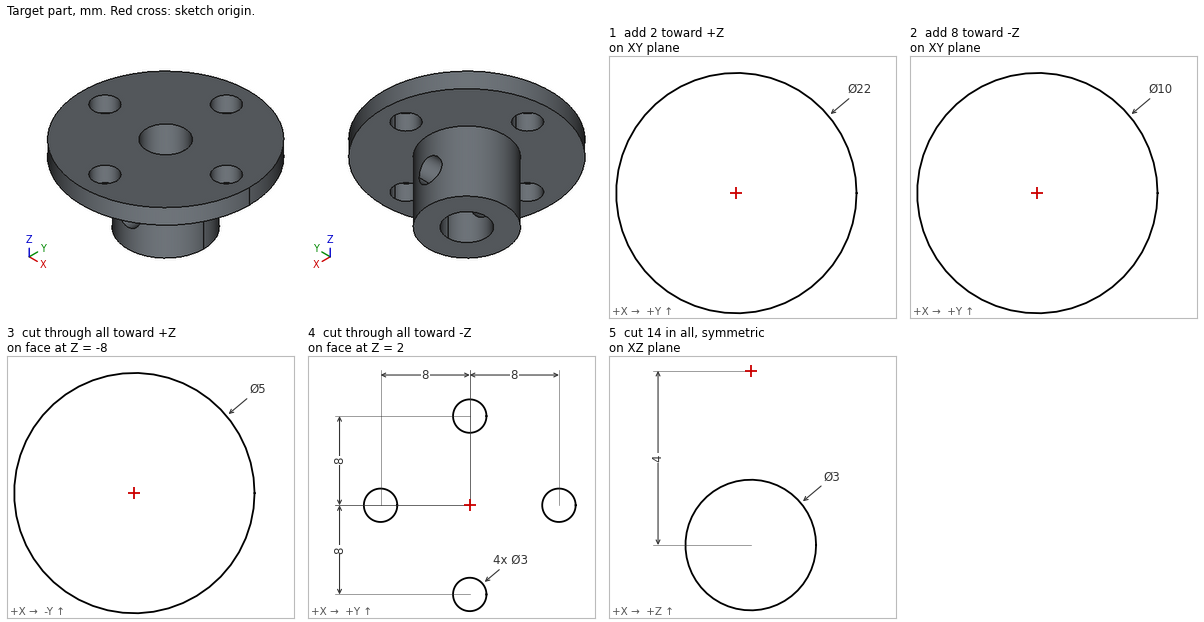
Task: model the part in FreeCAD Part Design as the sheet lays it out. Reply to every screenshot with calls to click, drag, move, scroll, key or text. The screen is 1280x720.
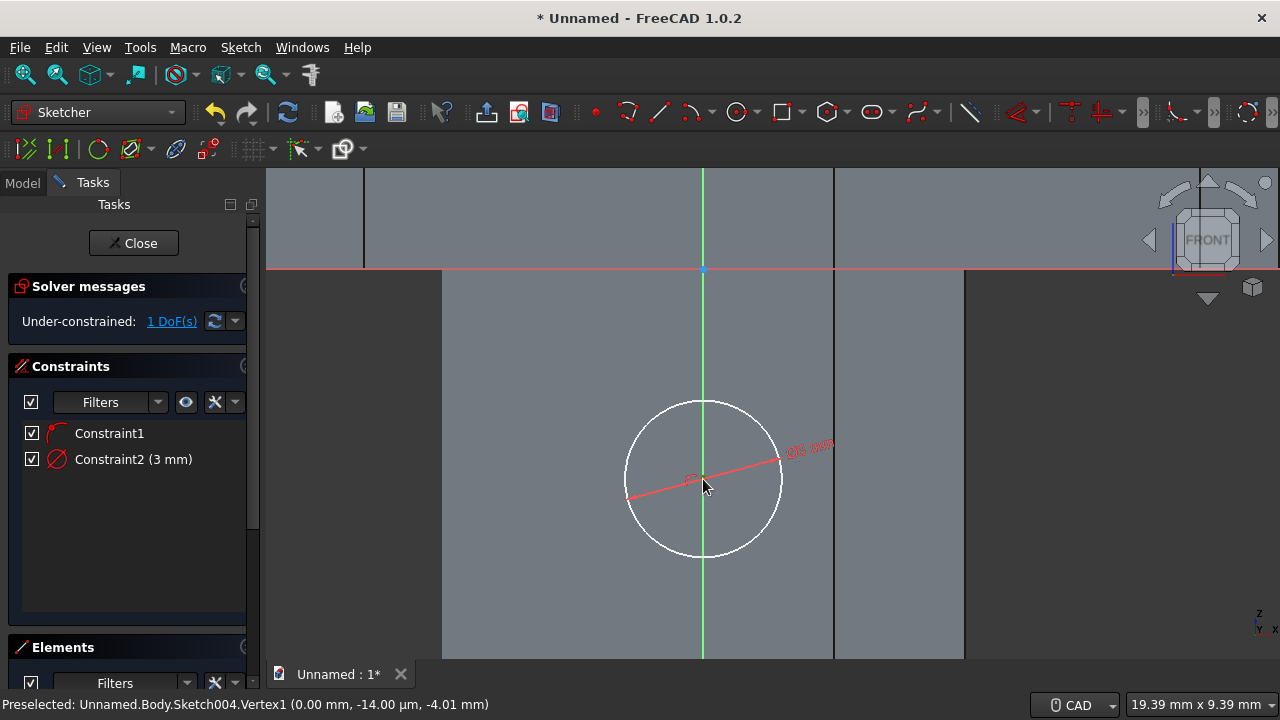
click(1038, 112)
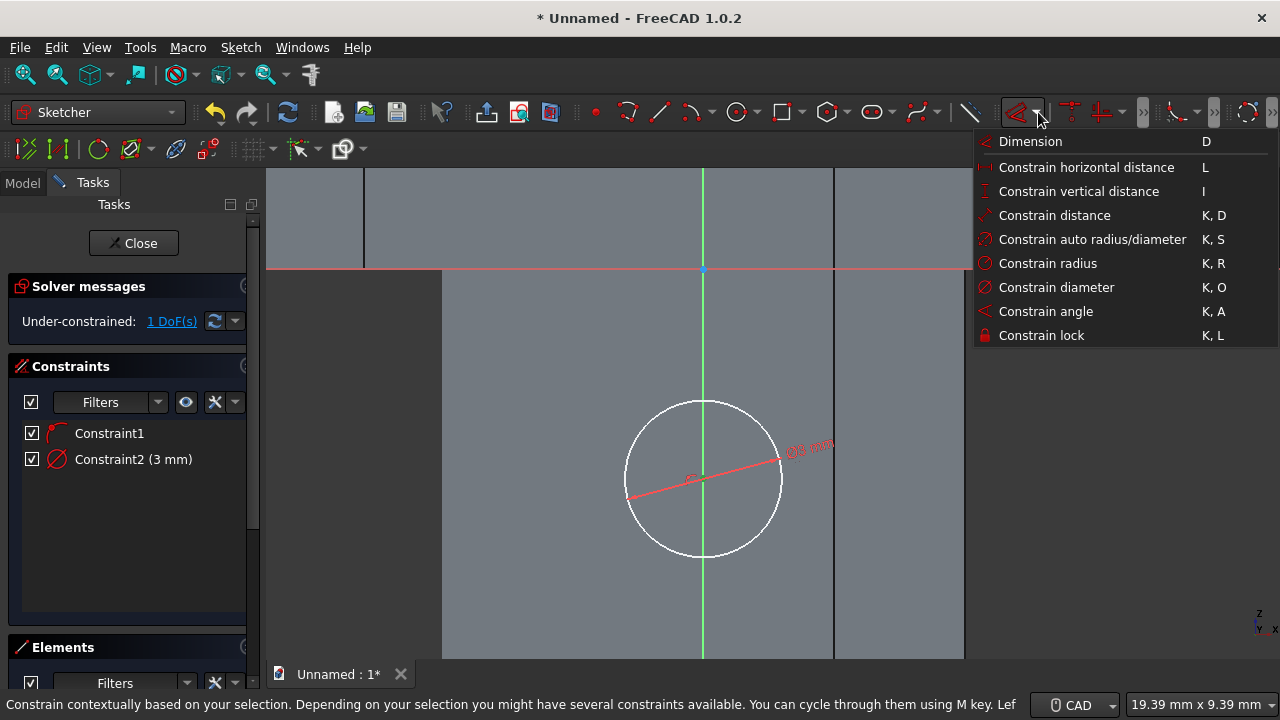
click(1126, 191)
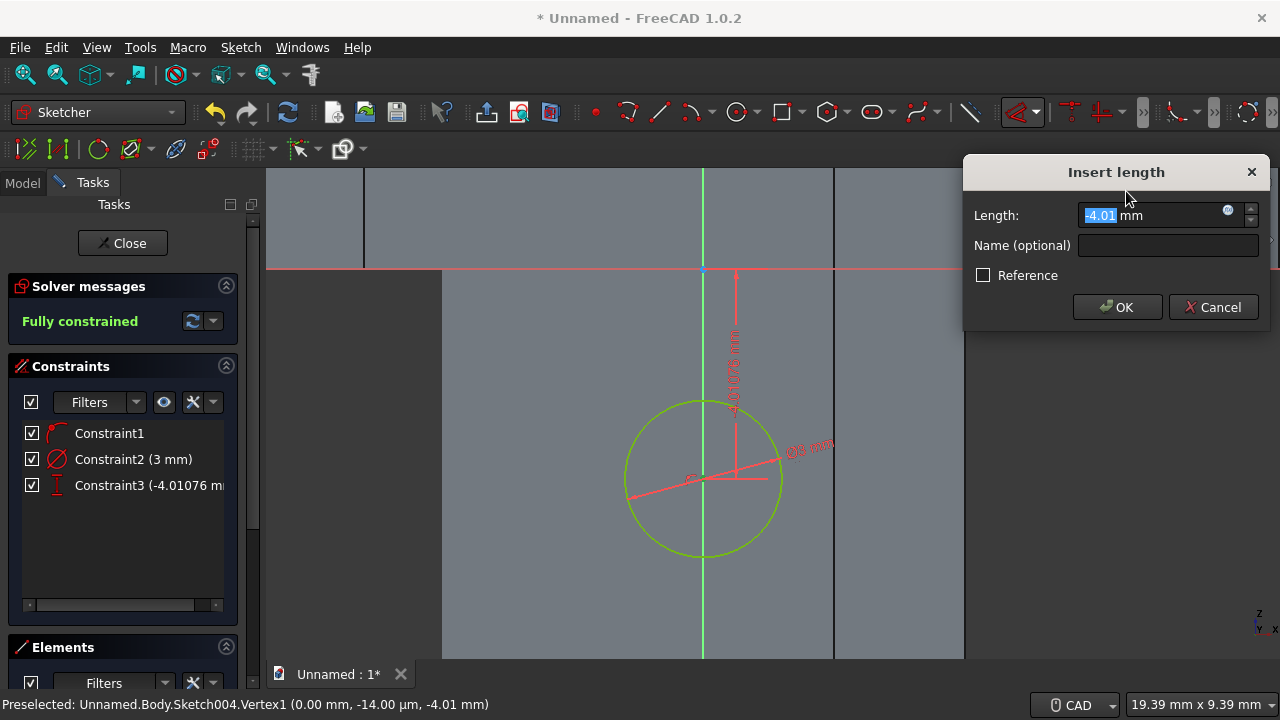
text(-4)
key(Return)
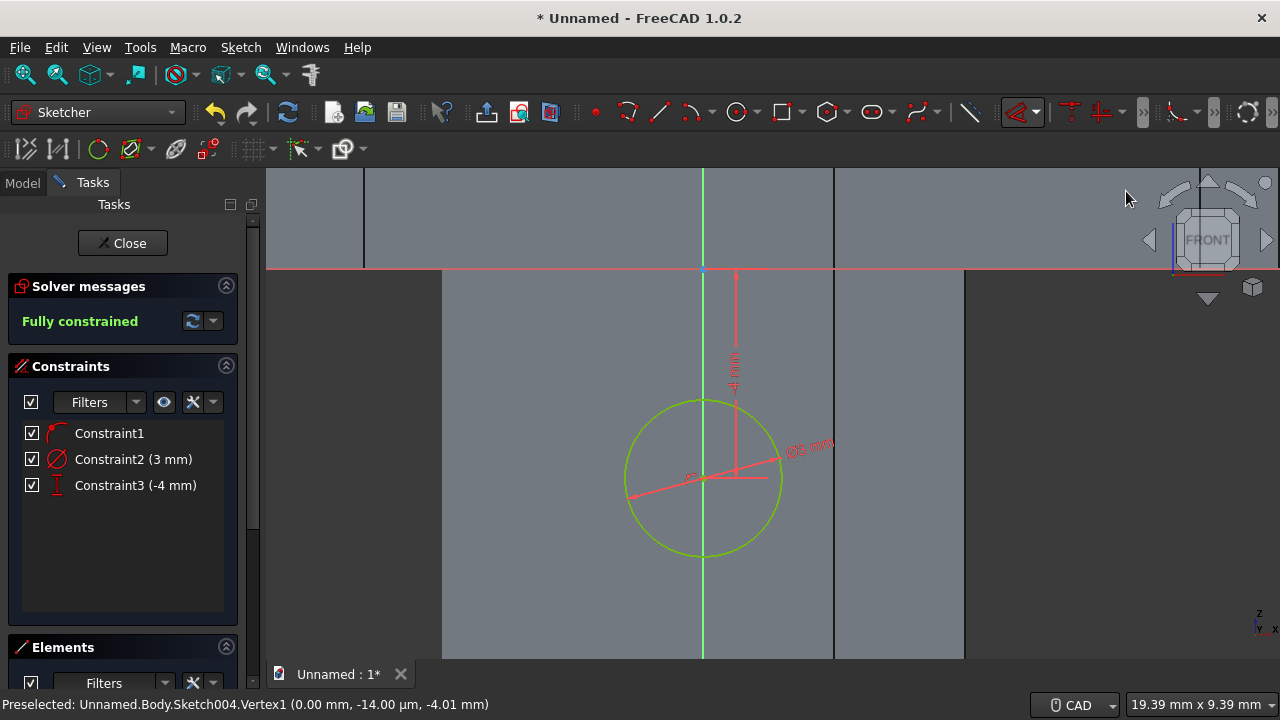
click(123, 243)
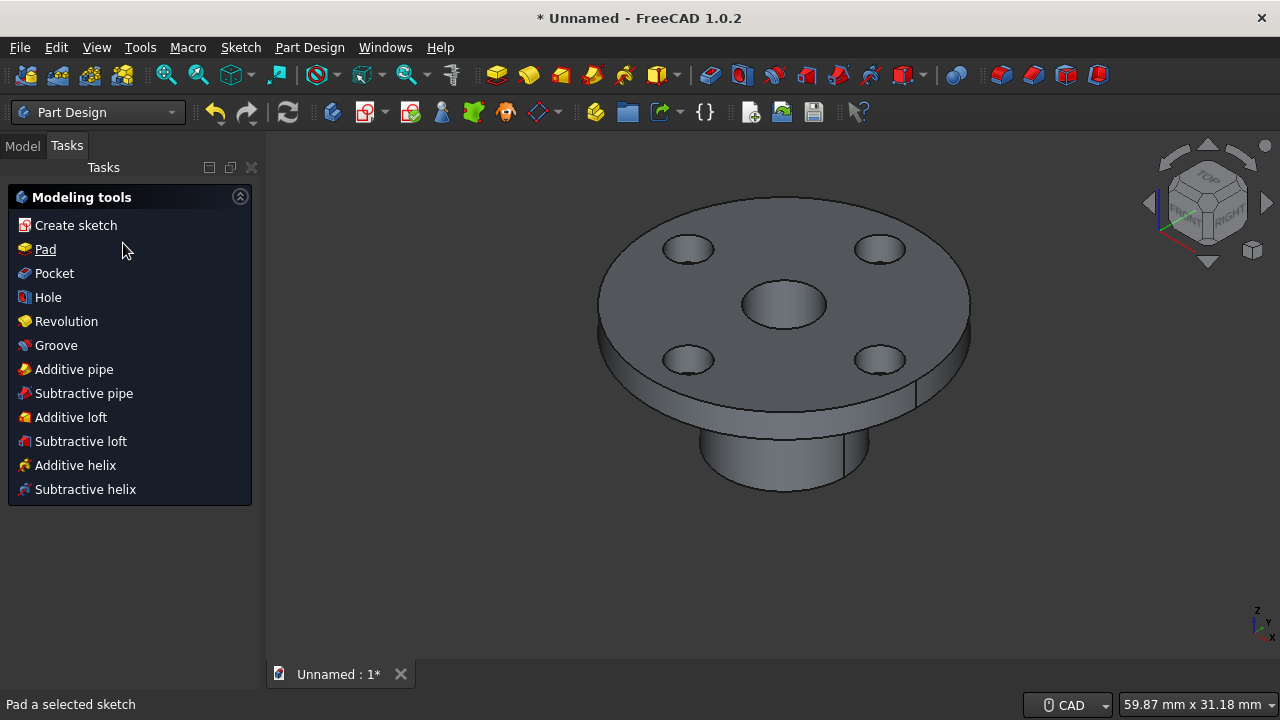
click(712, 76)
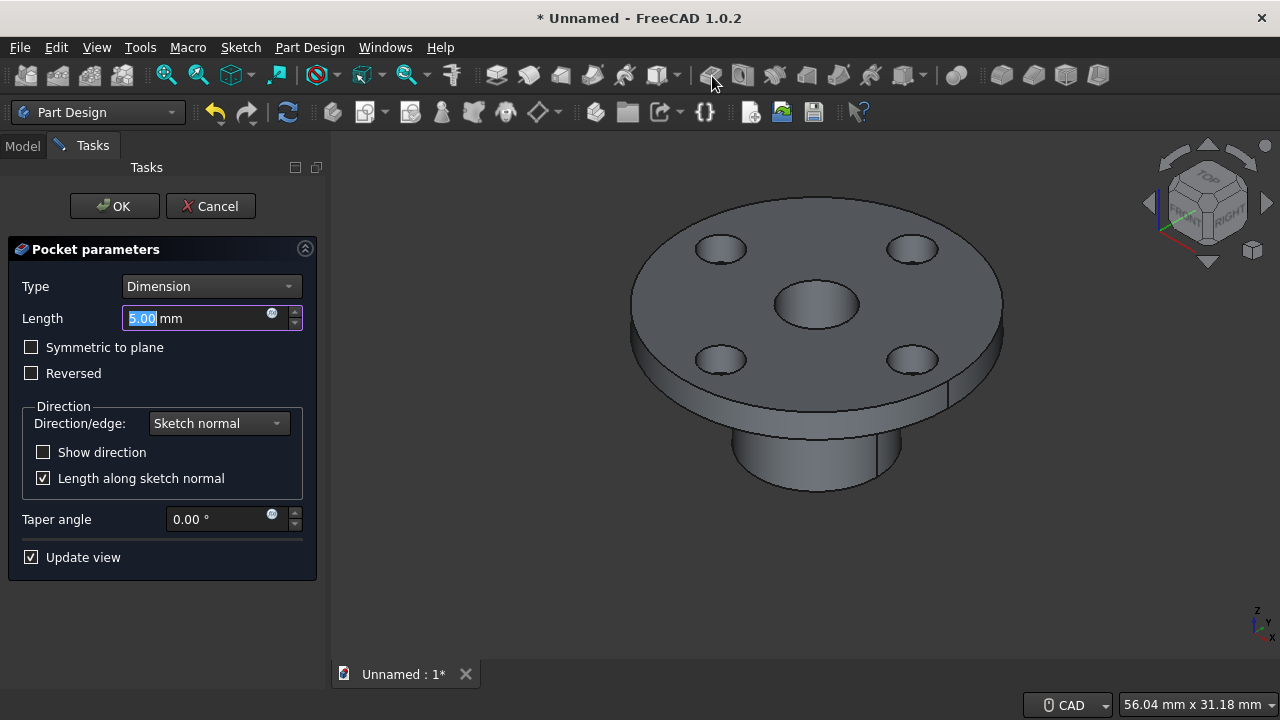
text(14)
key(Tab)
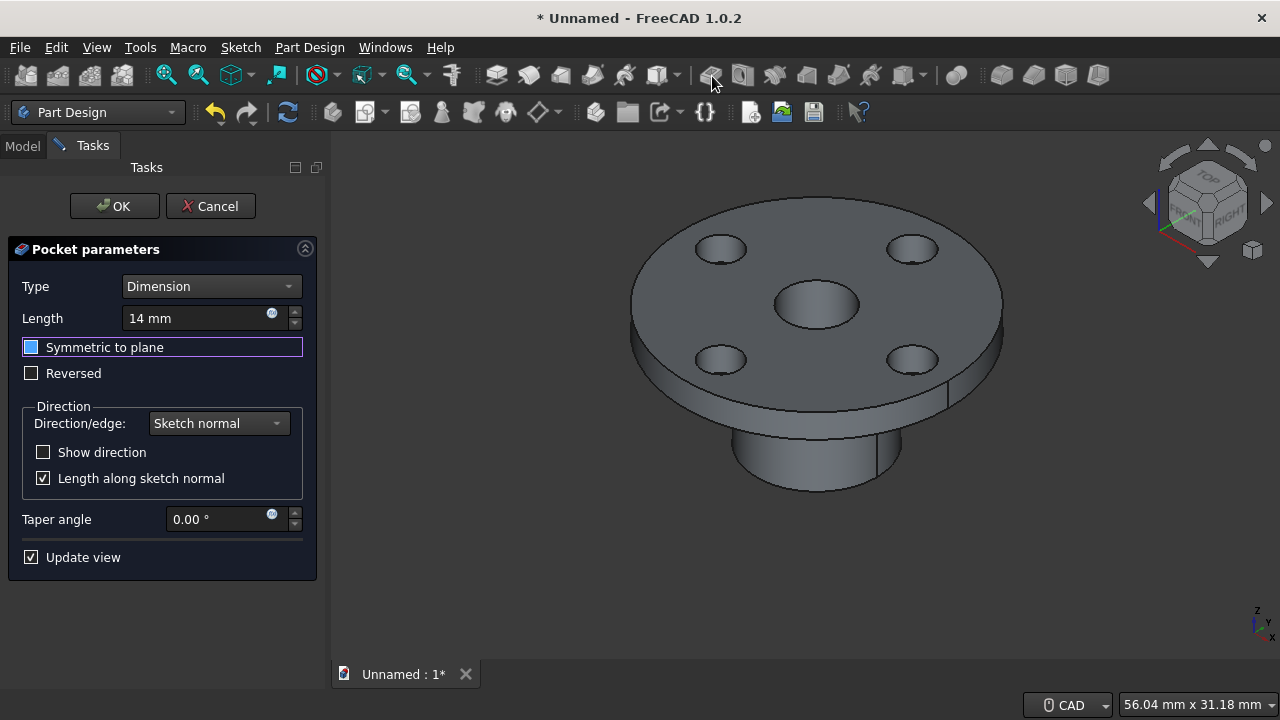
click(30, 347)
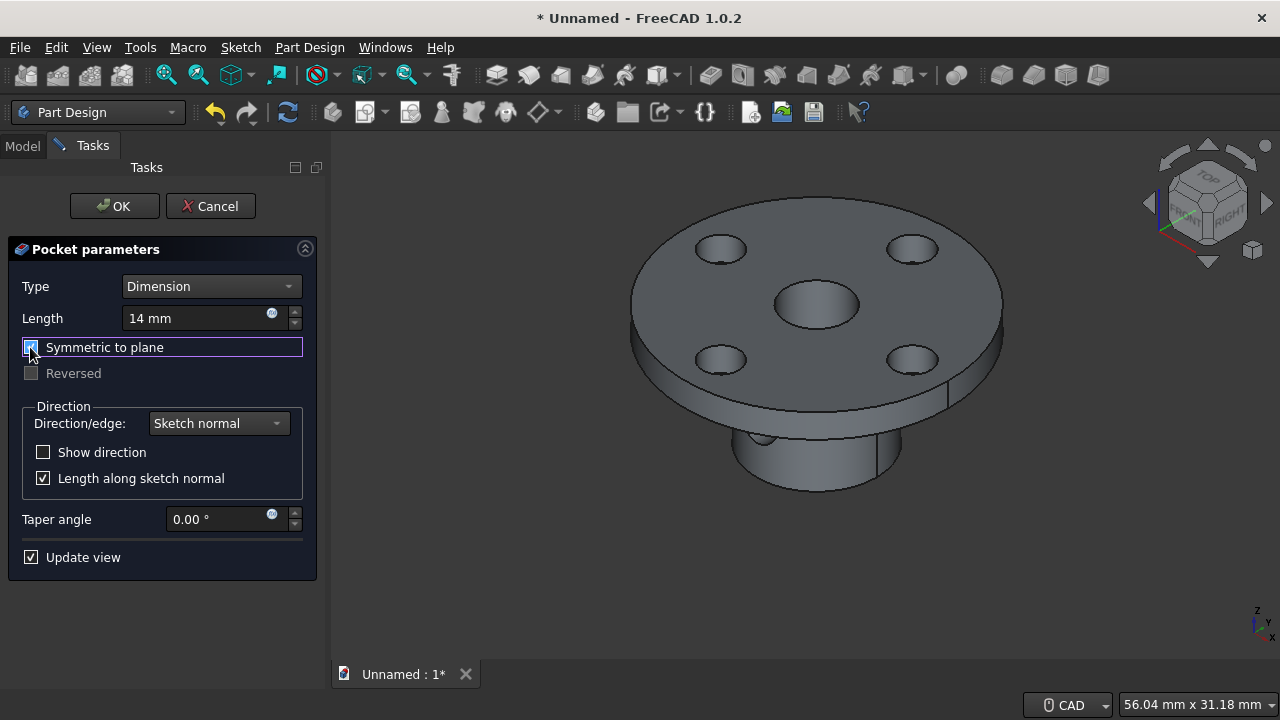
click(115, 206)